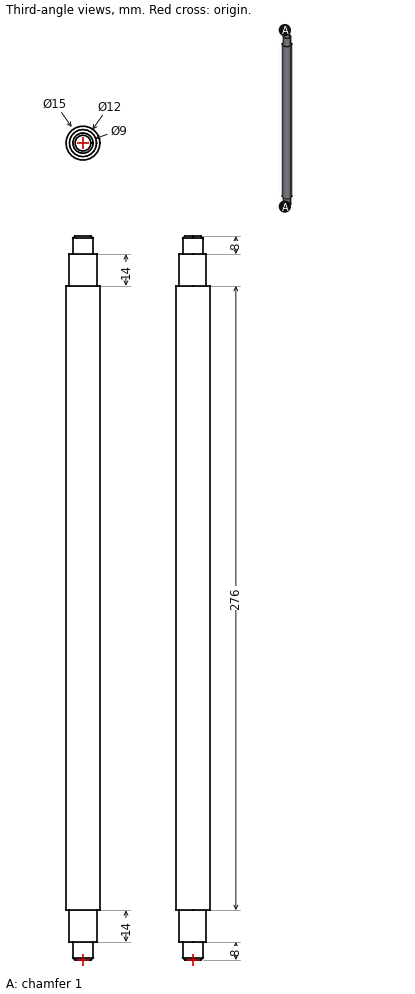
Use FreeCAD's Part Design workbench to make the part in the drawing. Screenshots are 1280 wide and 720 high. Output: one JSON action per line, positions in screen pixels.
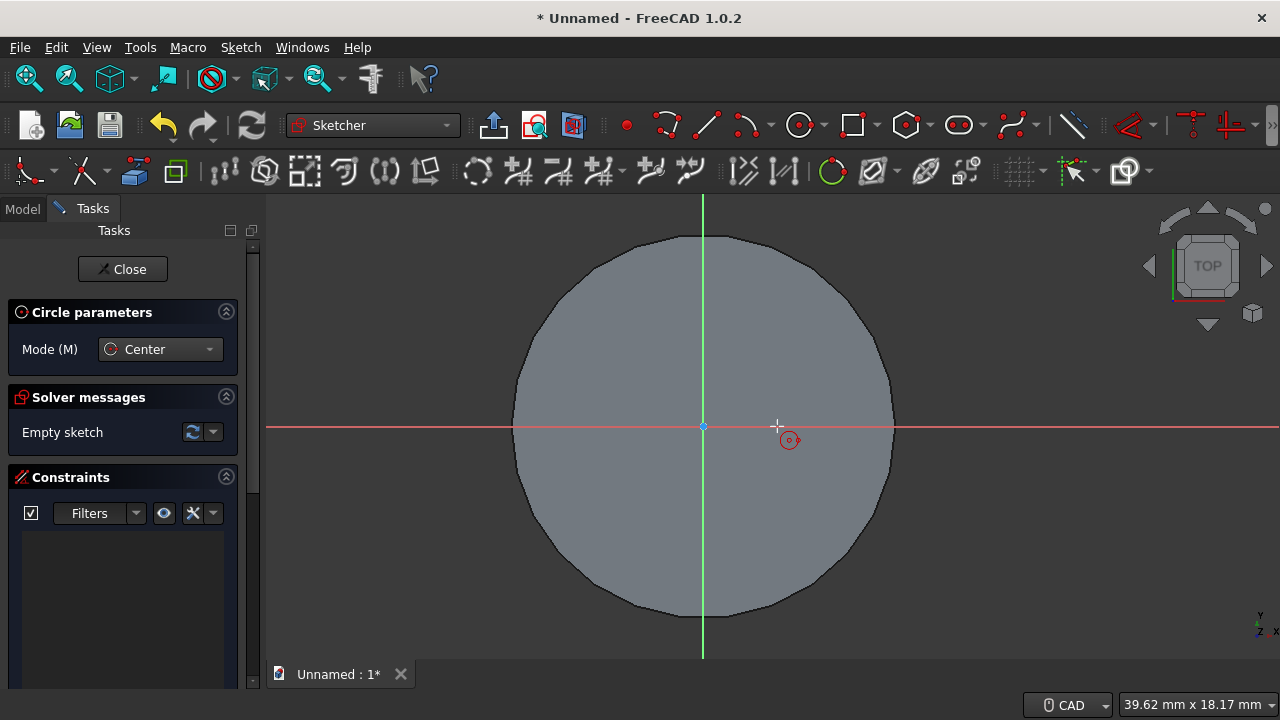
{"action": "left_click", "coordinate": [703, 426]}
{"action": "left_click", "coordinate": [812, 318]}
{"action": "key", "text": "Escape"}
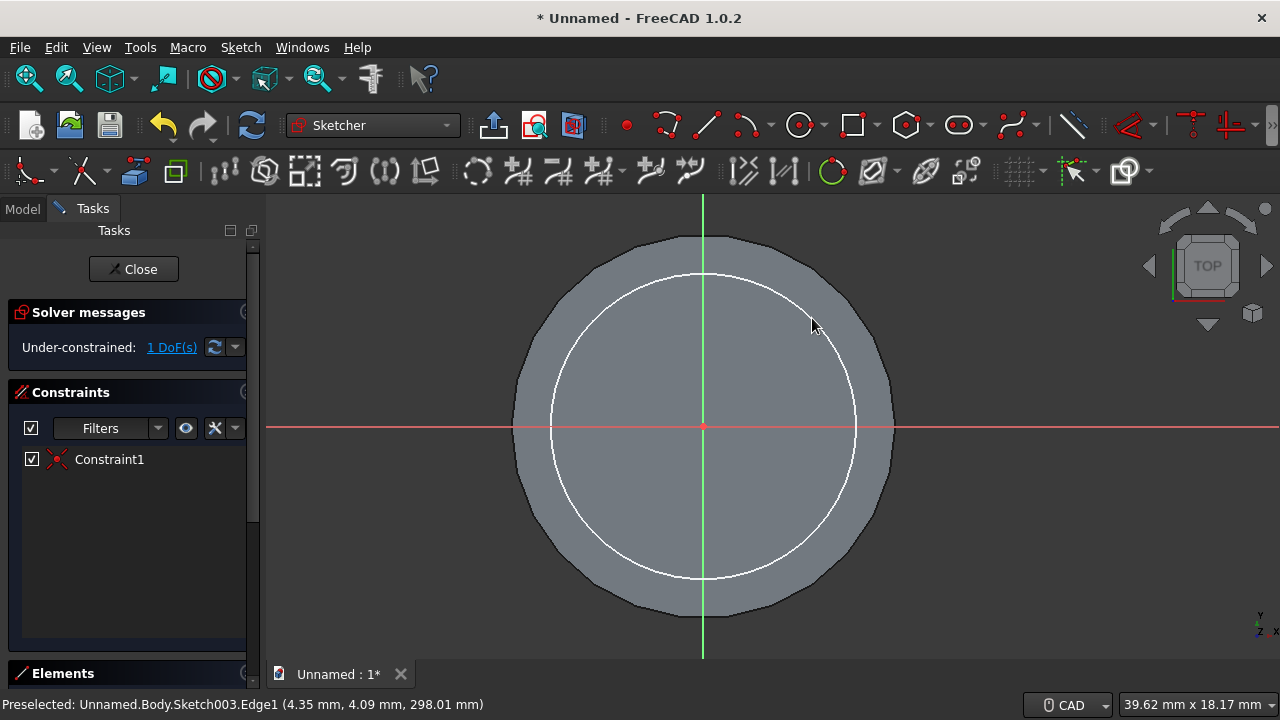
{"action": "left_click", "coordinate": [1128, 126]}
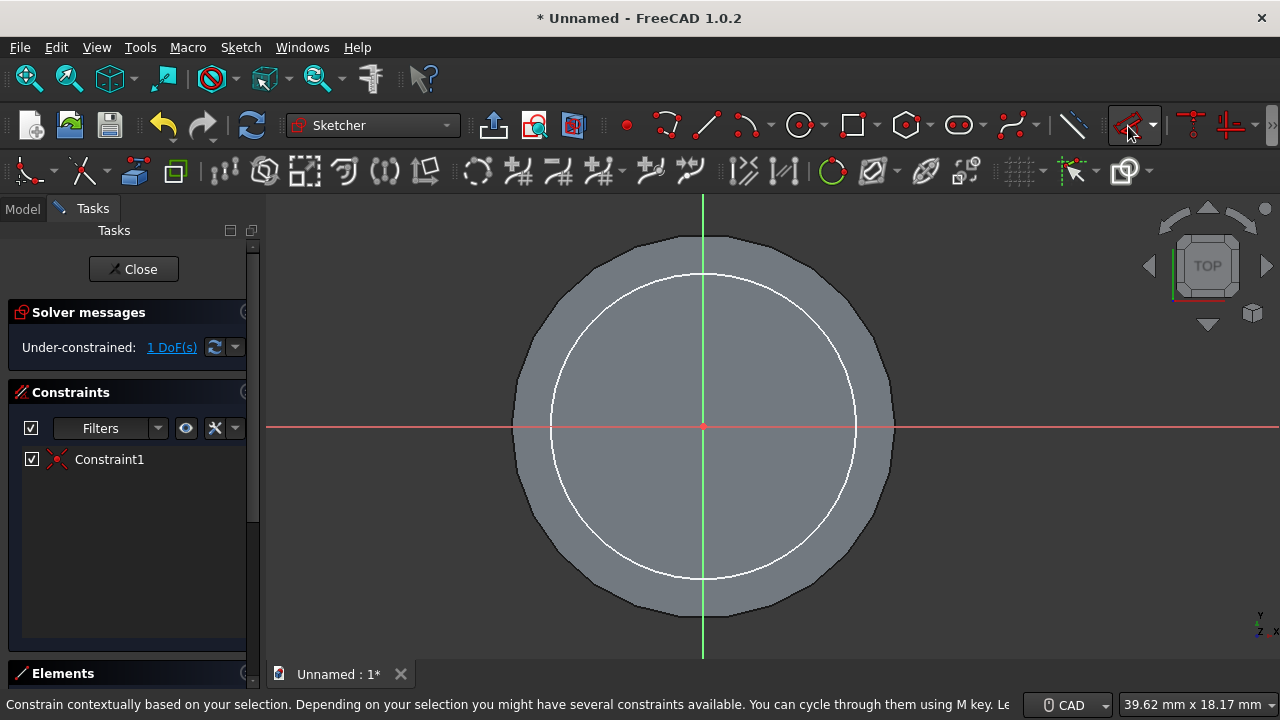
{"action": "left_click", "coordinate": [811, 318]}
{"action": "left_click", "coordinate": [834, 295]}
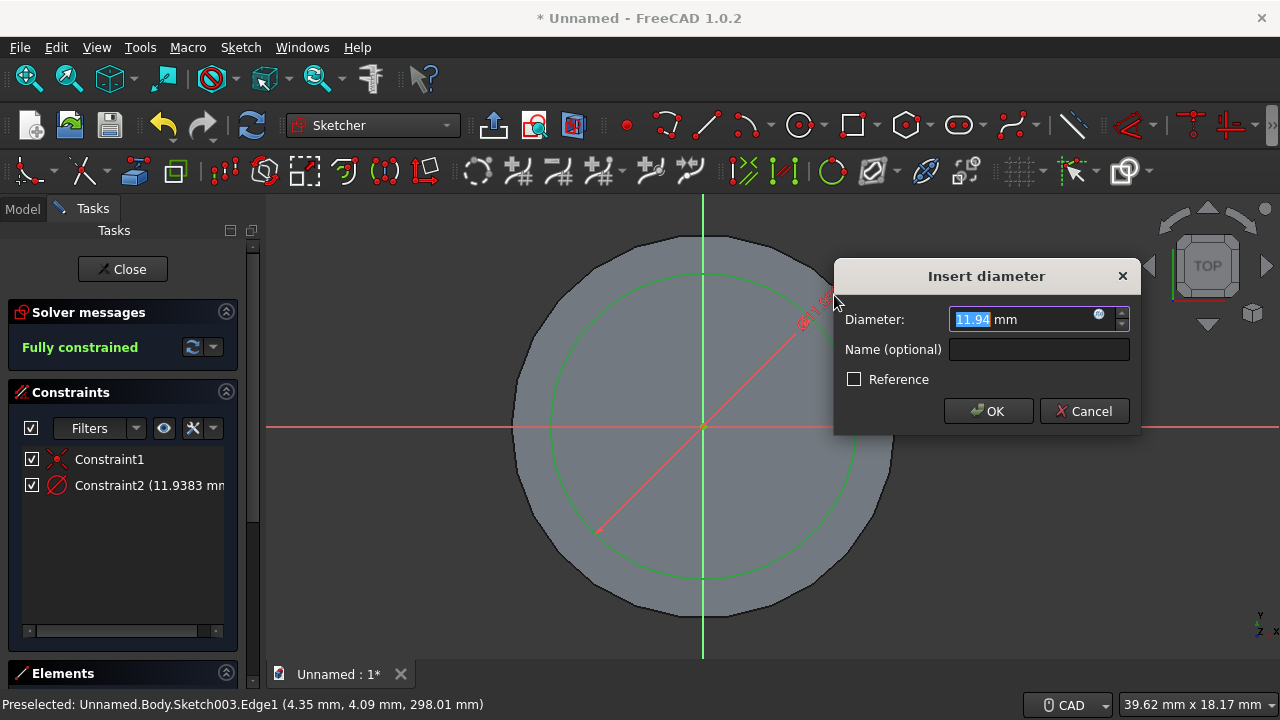
{"action": "type", "text": "12"}
{"action": "key", "text": "Return"}
{"action": "key", "text": "Escape"}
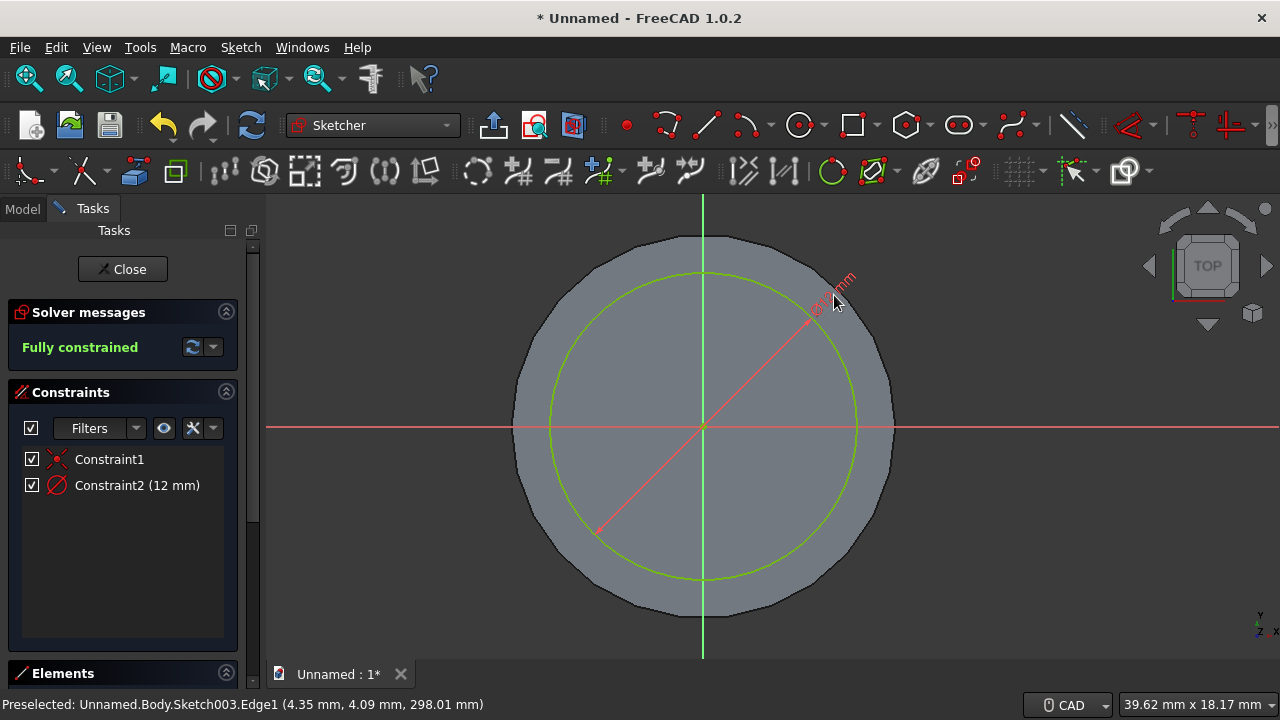
{"action": "left_click", "coordinate": [123, 269]}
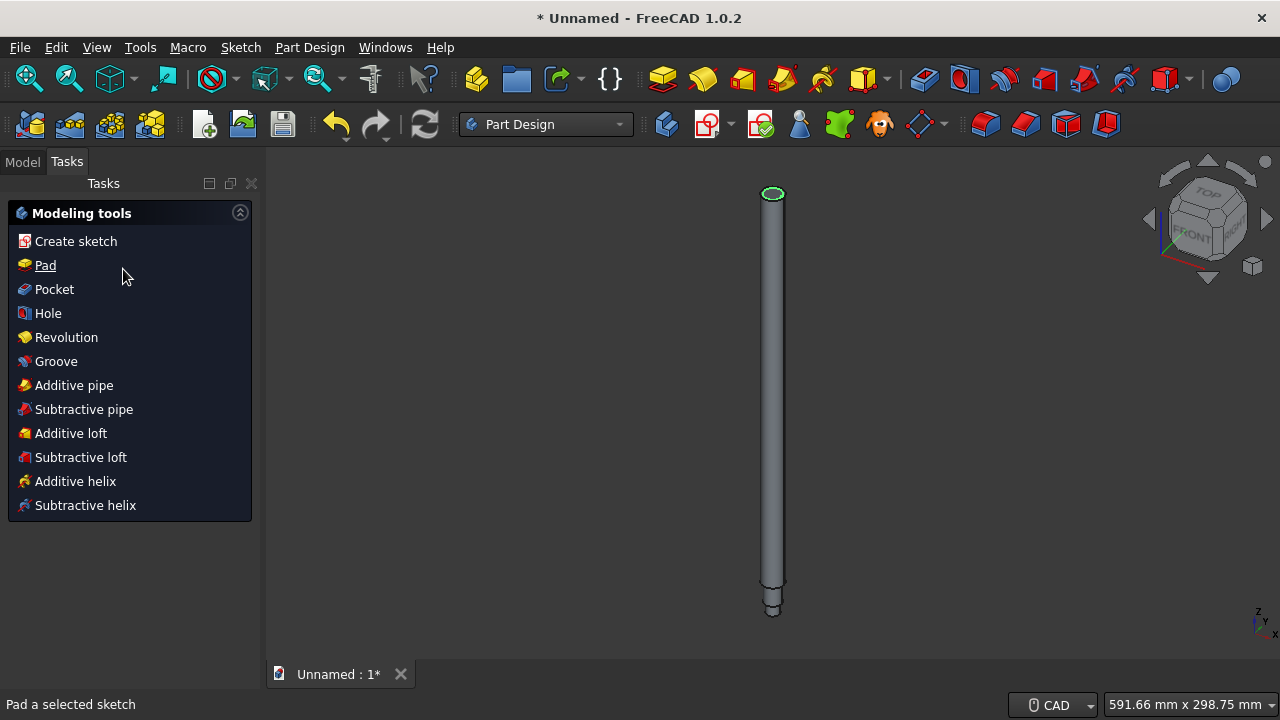
{"action": "left_click", "coordinate": [664, 80]}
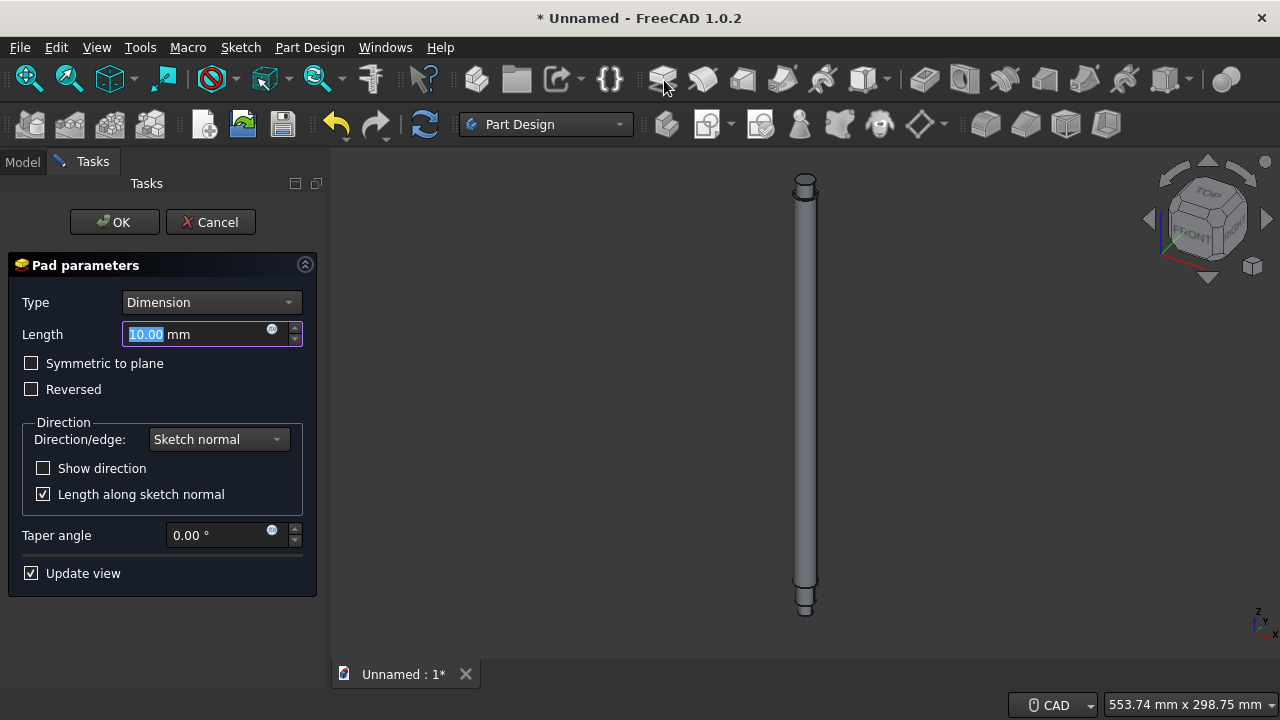
{"action": "type", "text": "14"}
{"action": "key", "text": "Tab"}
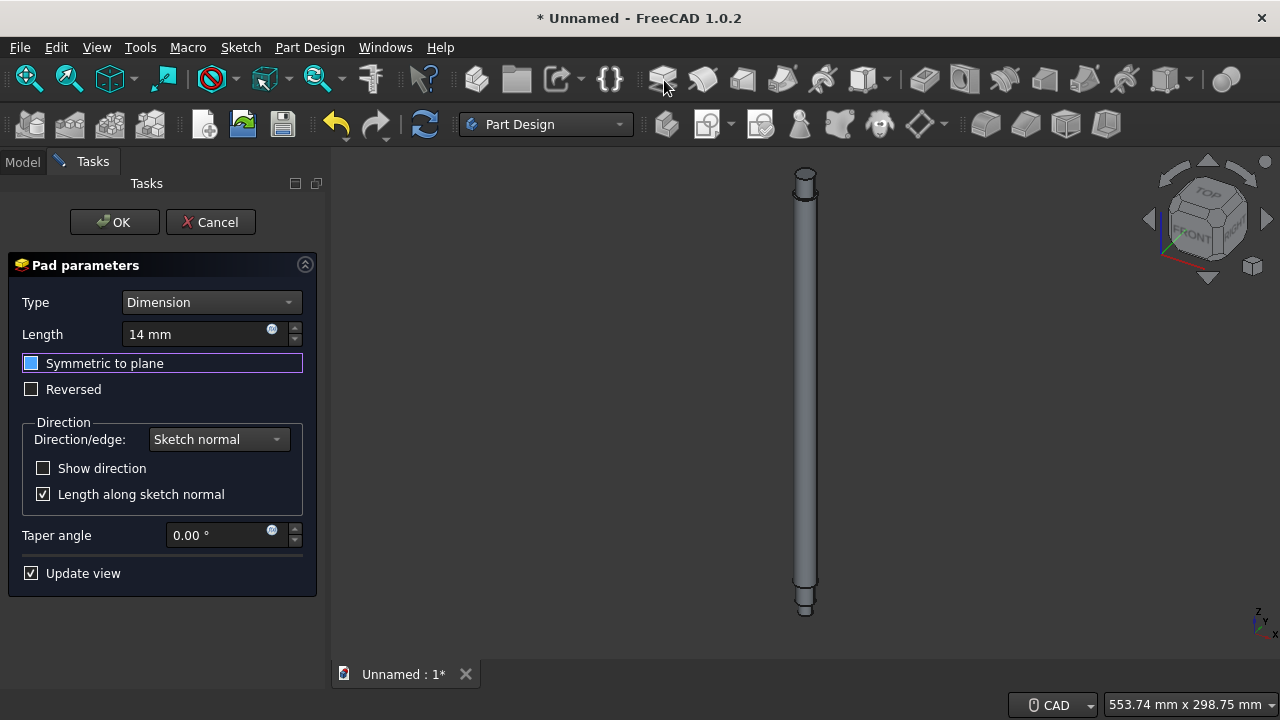
{"action": "left_click", "coordinate": [115, 222]}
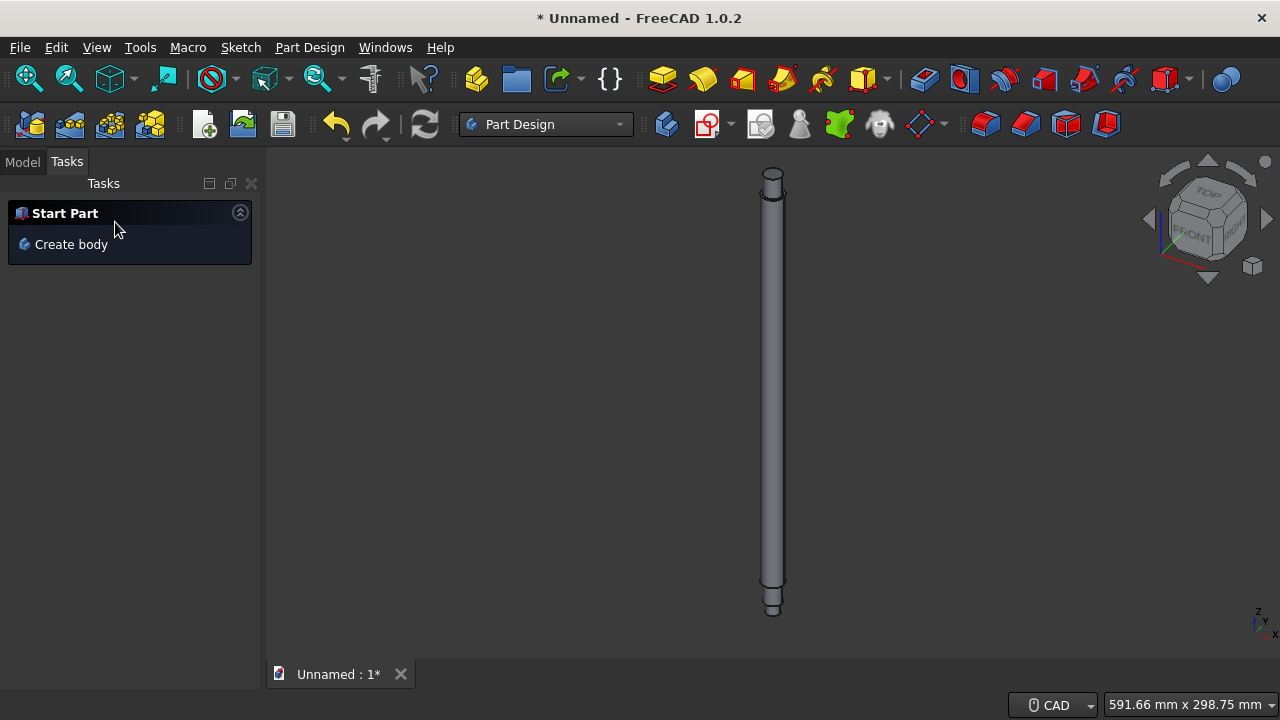
{"action": "key", "text": "0"}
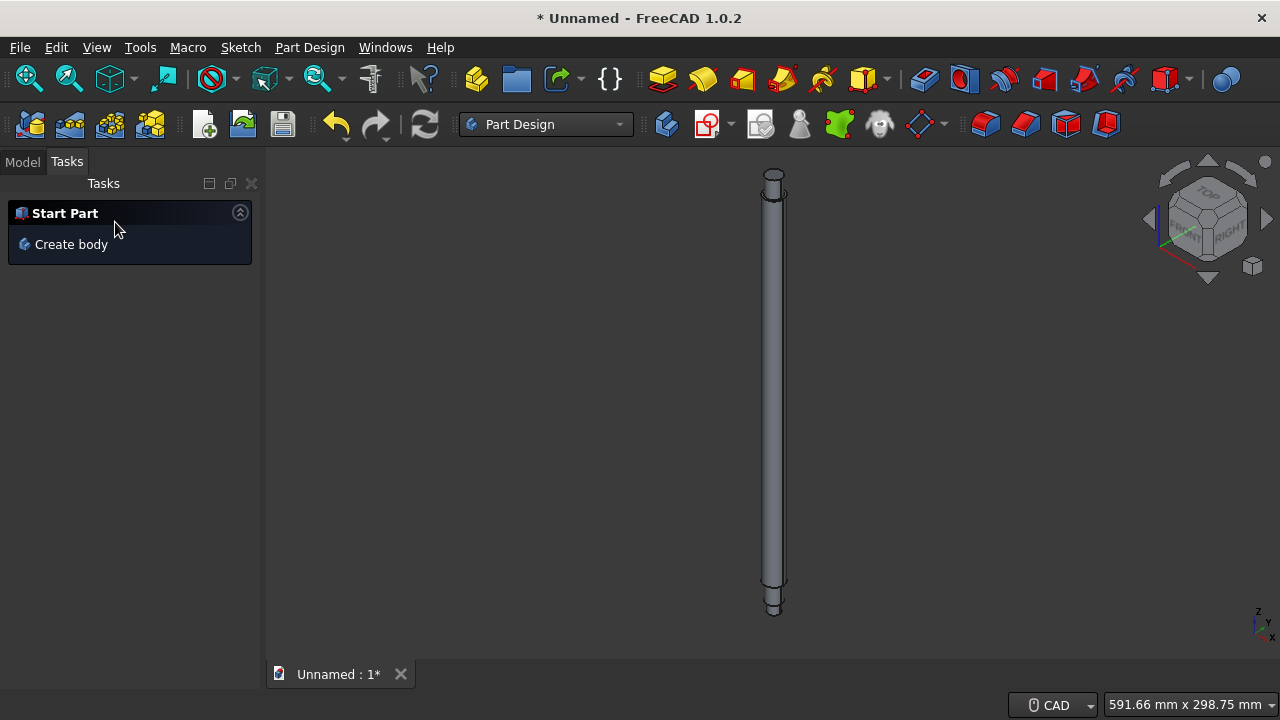
{"action": "key", "text": "2"}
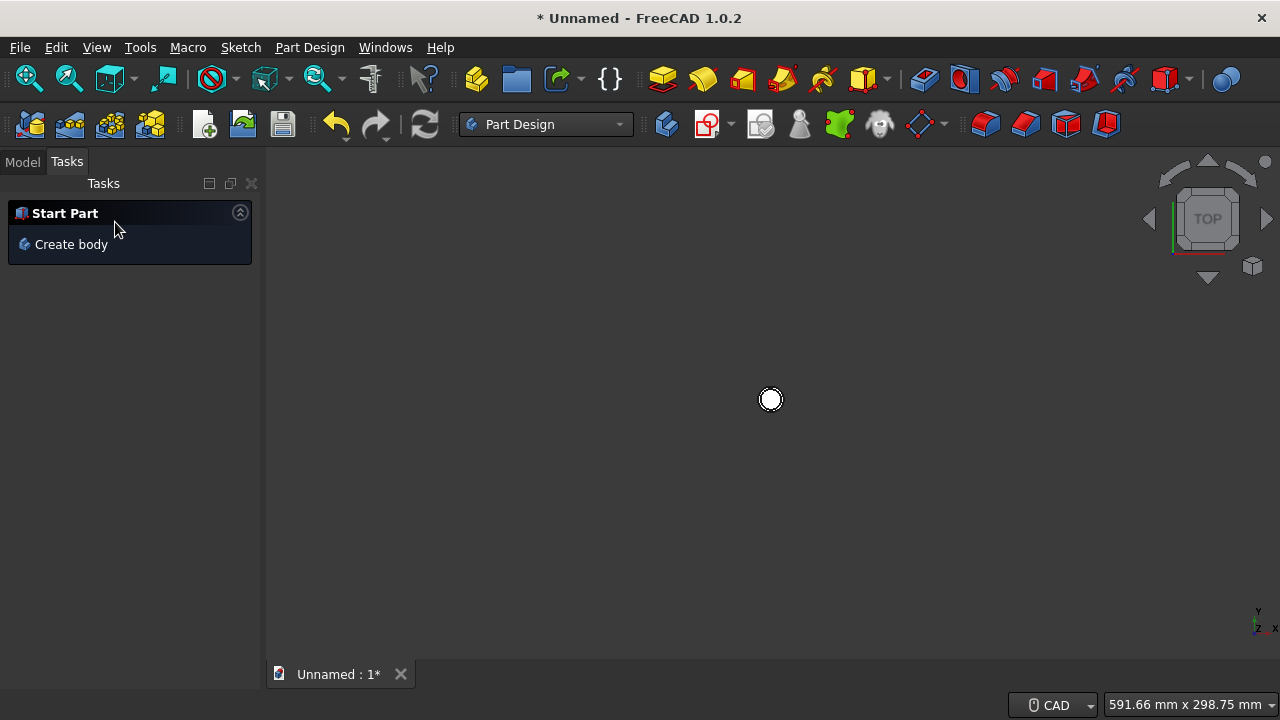
{"action": "key", "text": "v f"}